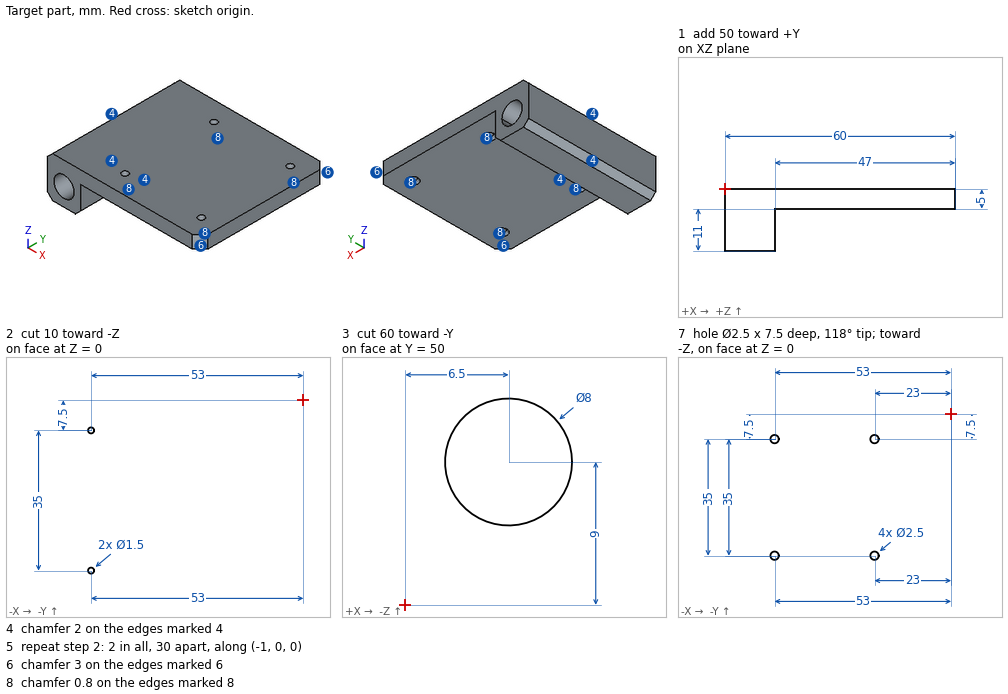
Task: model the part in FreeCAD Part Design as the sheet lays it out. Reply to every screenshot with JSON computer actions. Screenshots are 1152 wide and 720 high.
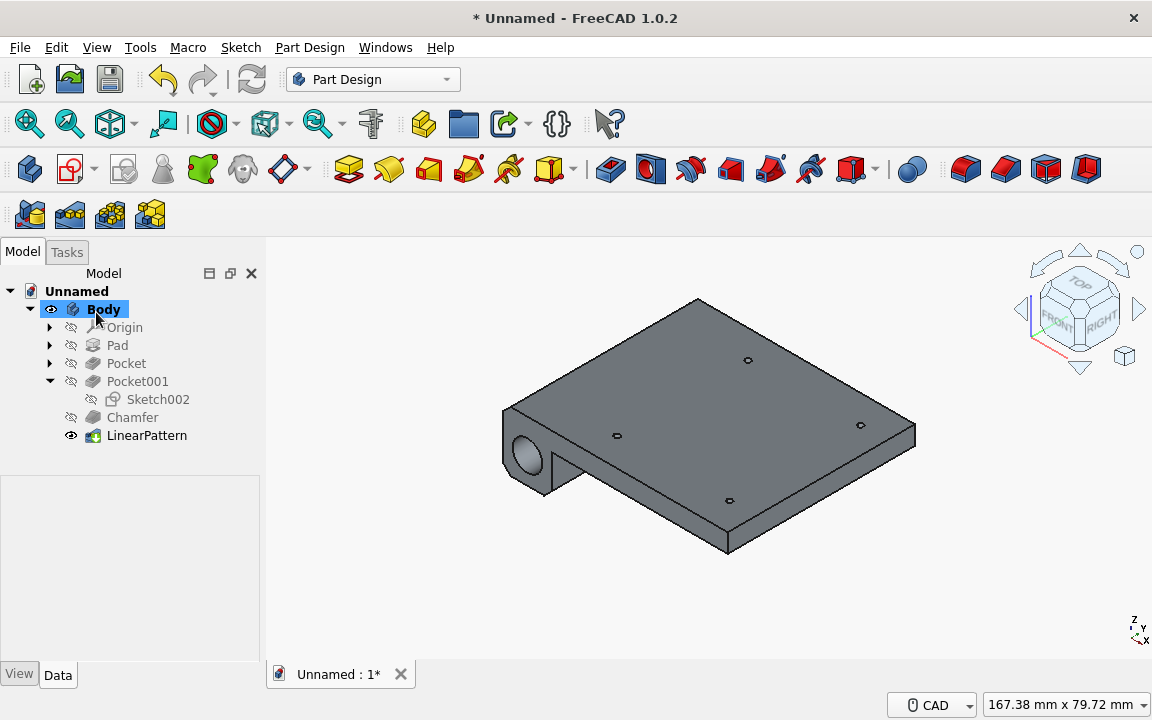
{"action": "left_click", "coordinate": [728, 542]}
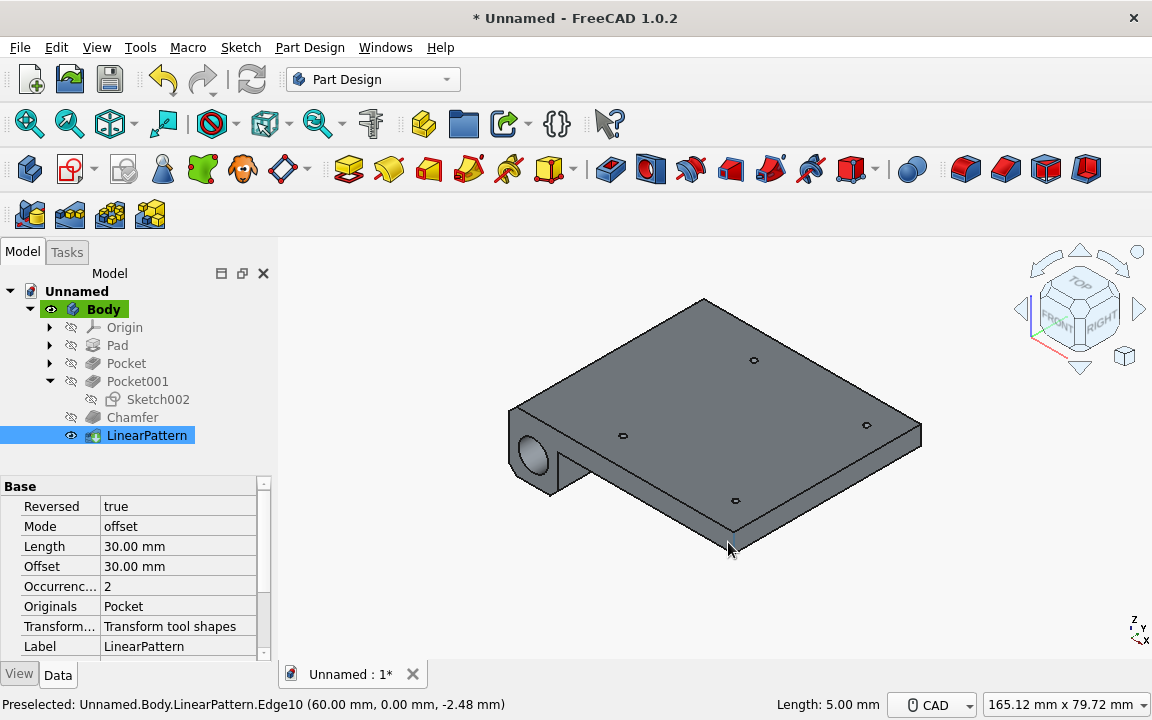
{"action": "key", "text": "2"}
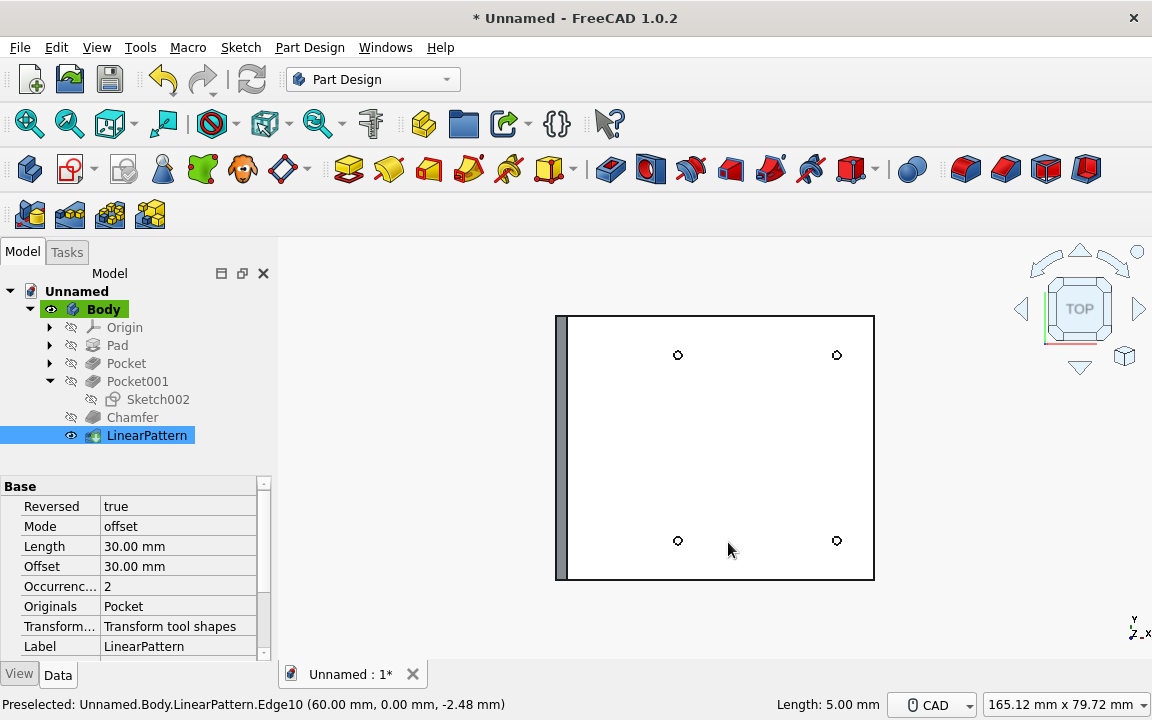
{"action": "key", "text": "0"}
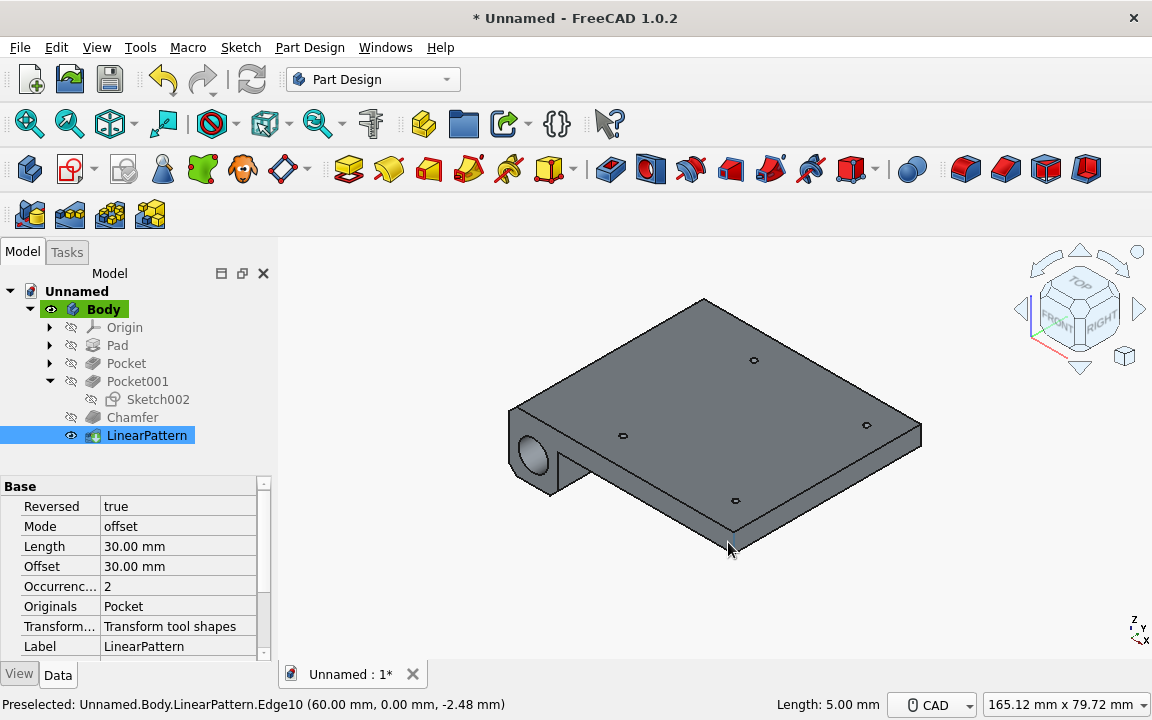
{"action": "key", "text": "1"}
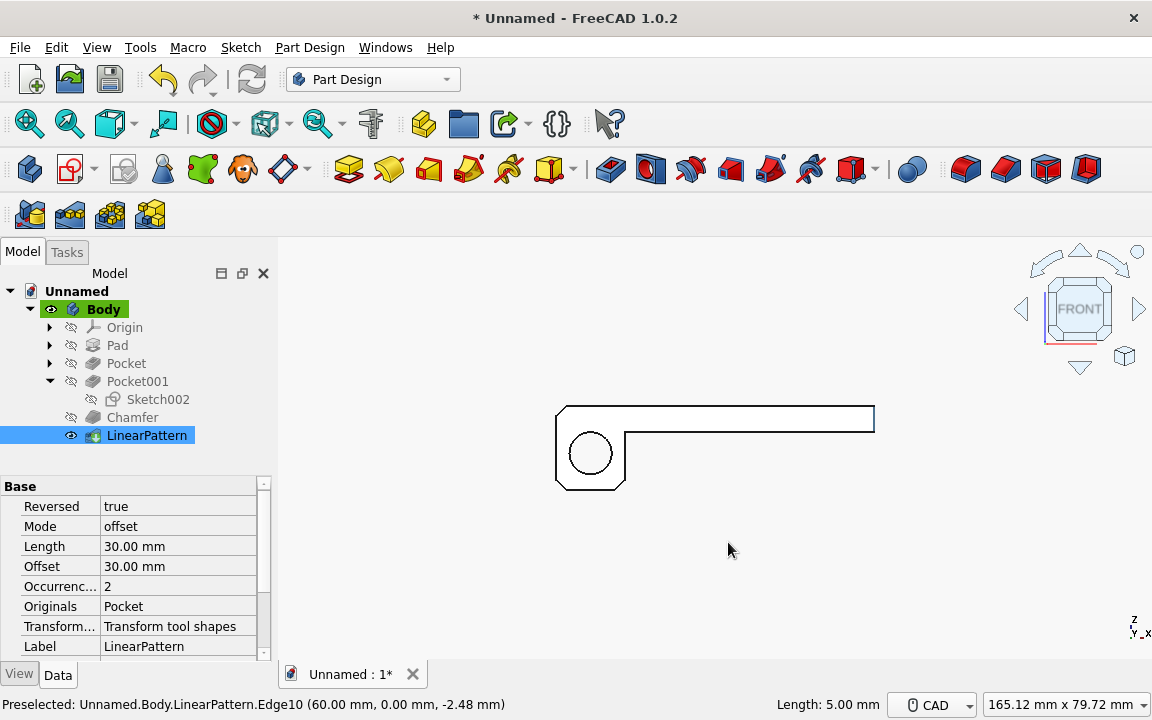
{"action": "left_click", "coordinate": [30, 124]}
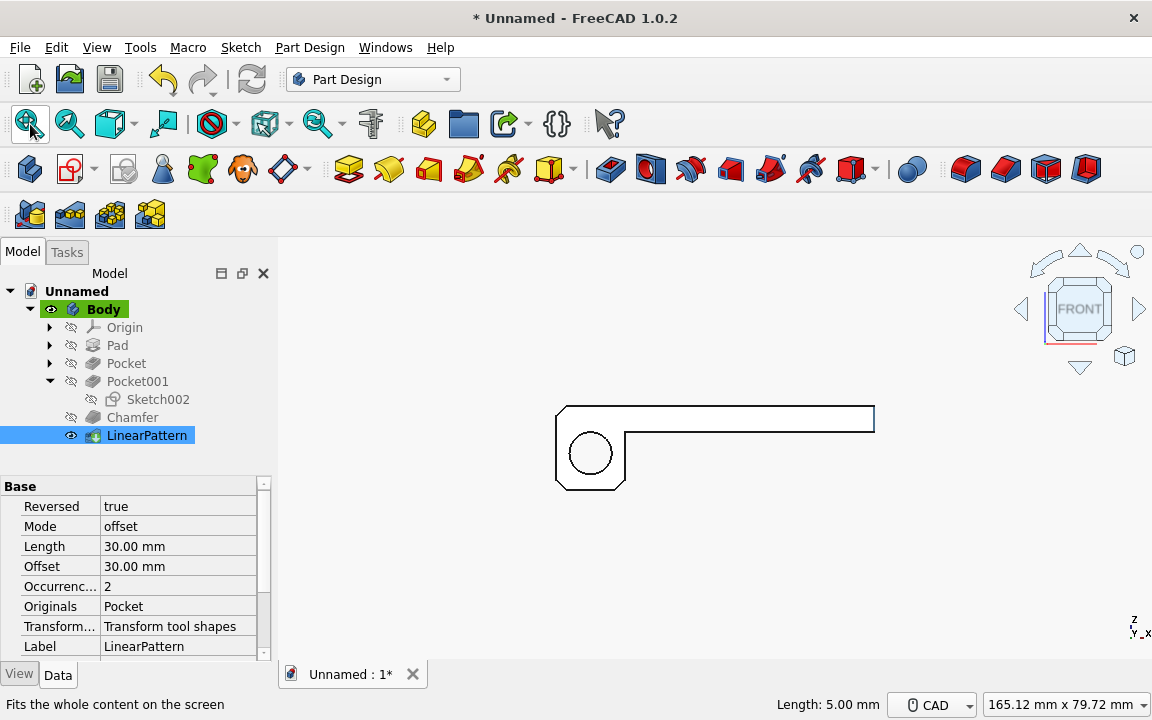
{"action": "key", "text": "3"}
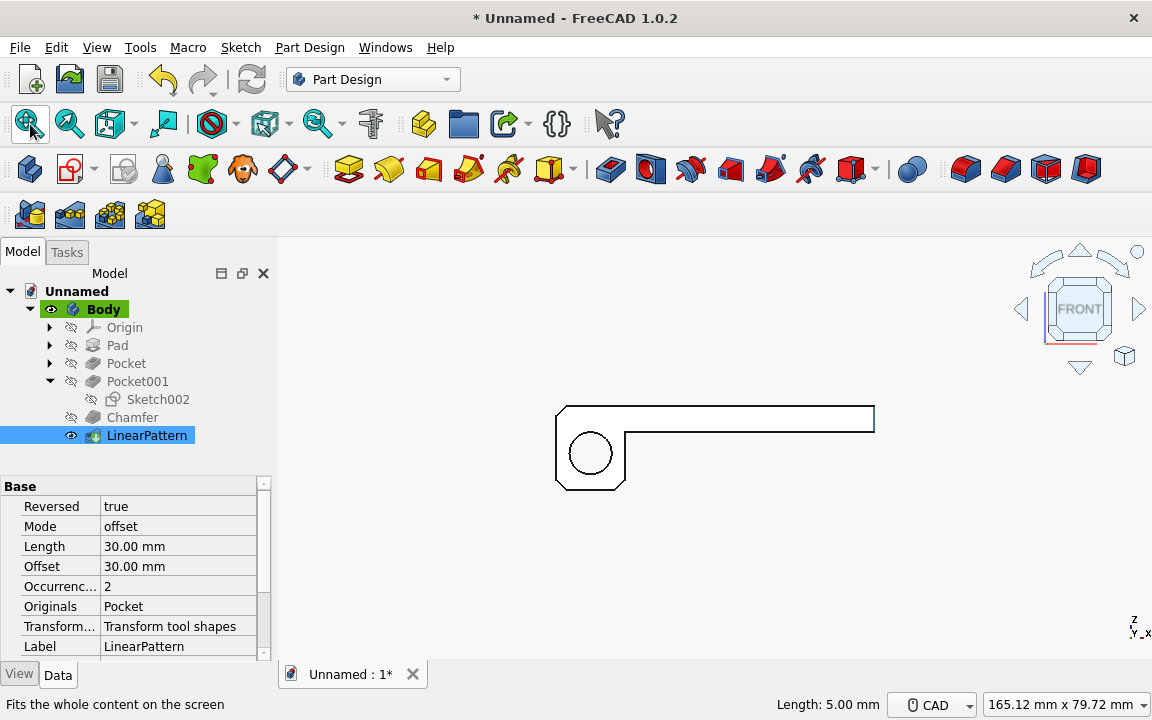
{"action": "left_click", "coordinate": [30, 124]}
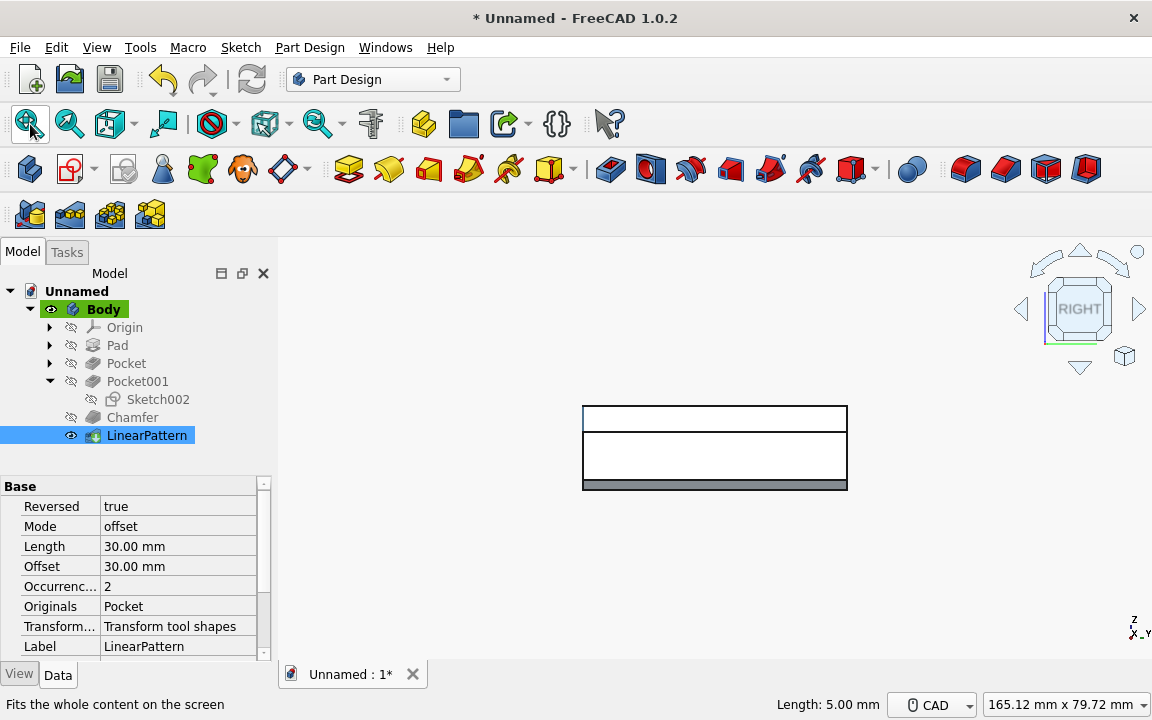
{"action": "left_click", "coordinate": [847, 418], "text": "ctrl"}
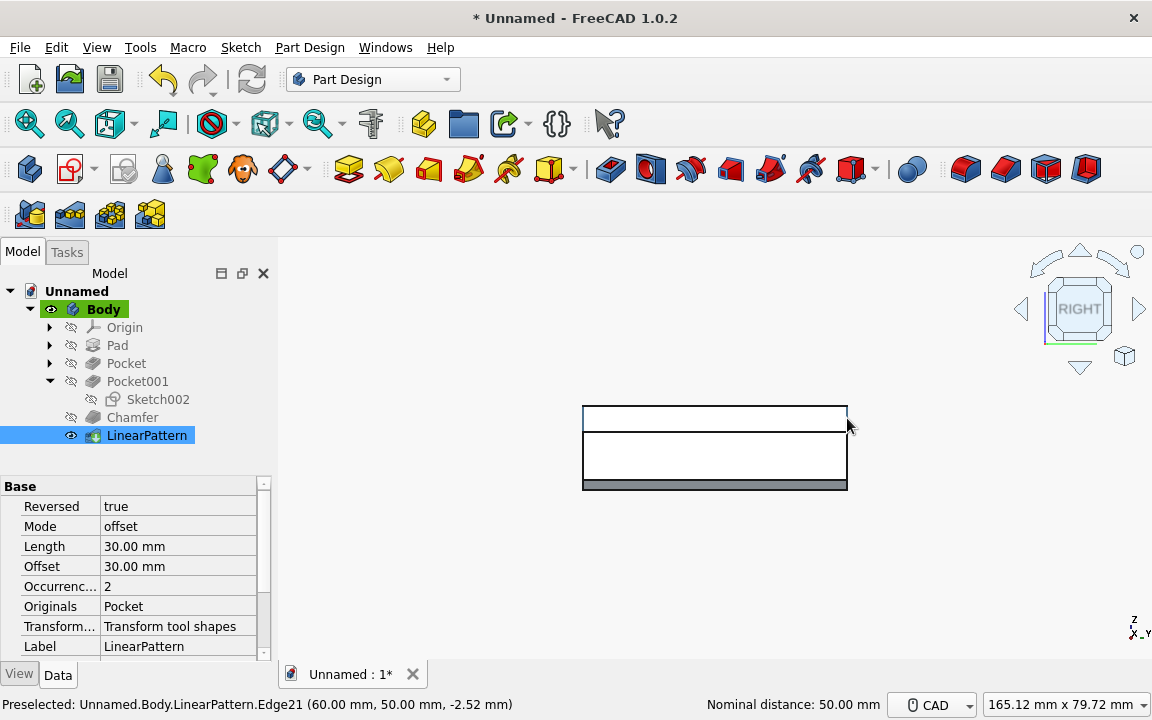
{"action": "left_click", "coordinate": [1006, 170]}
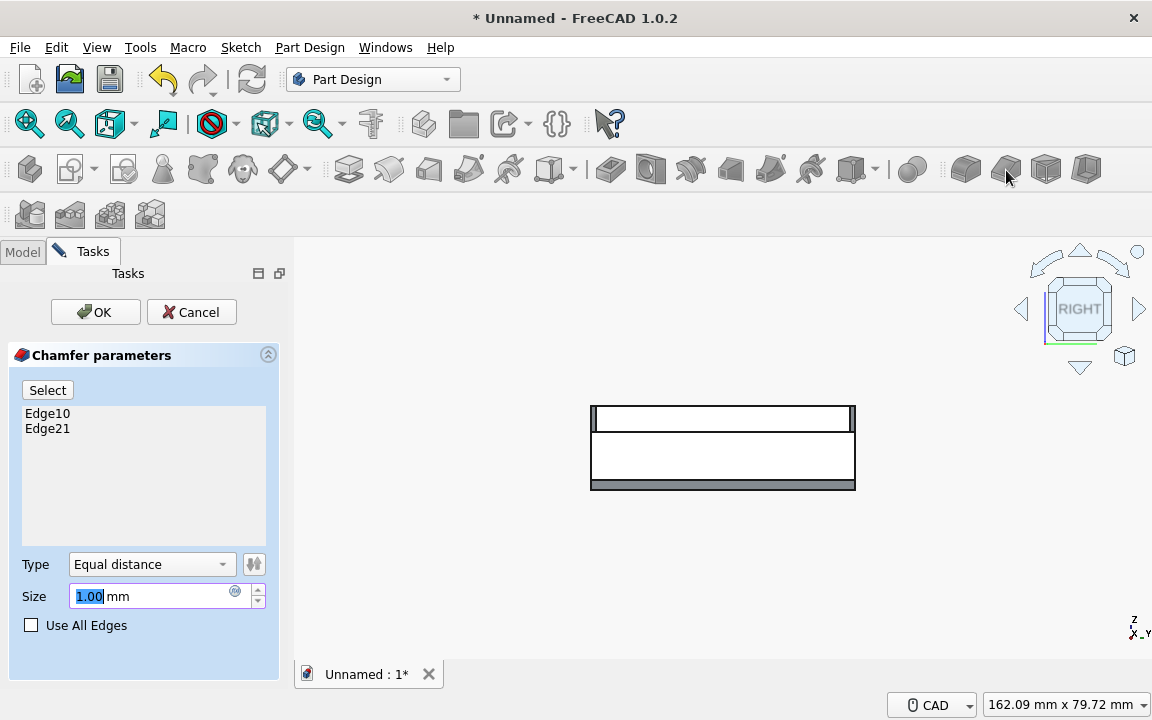
{"action": "type", "text": "3"}
{"action": "key", "text": "Tab"}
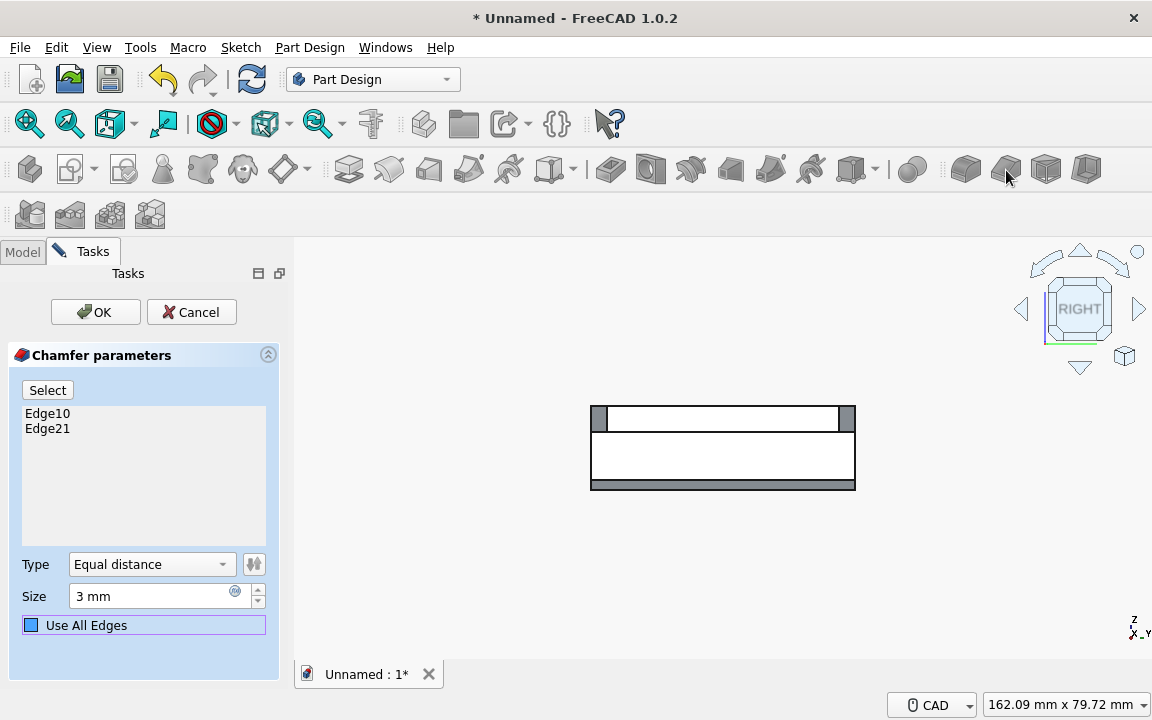
{"action": "left_click", "coordinate": [96, 312]}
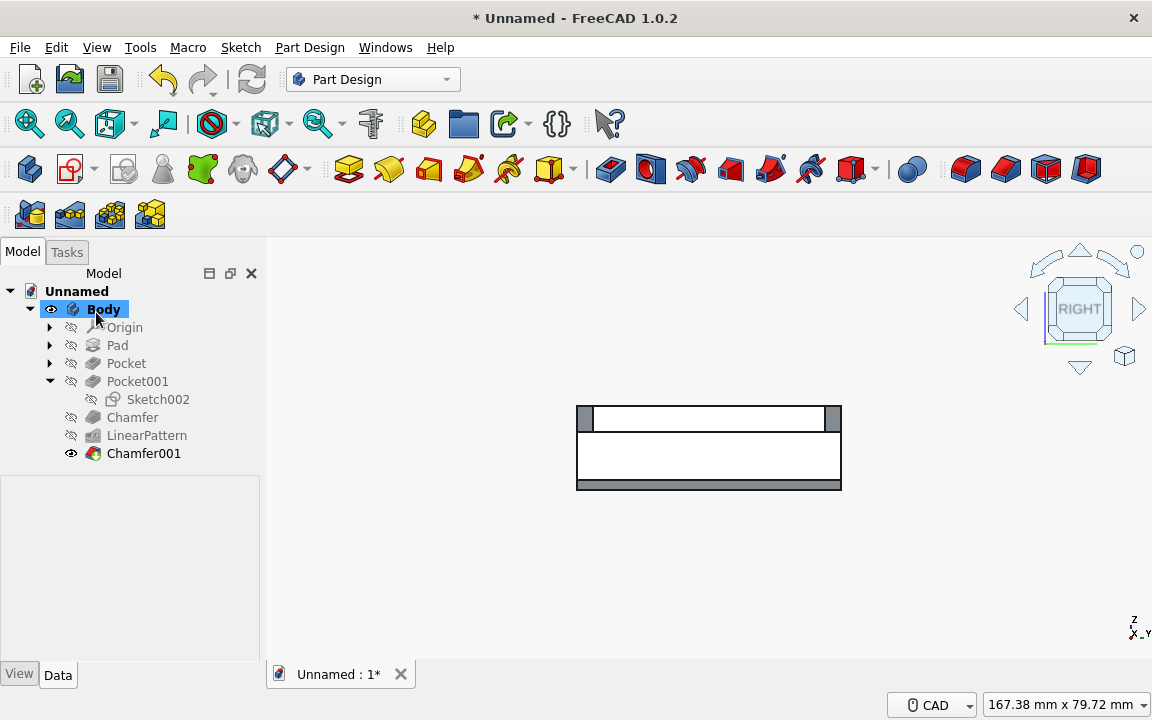
{"action": "left_click", "coordinate": [30, 124]}